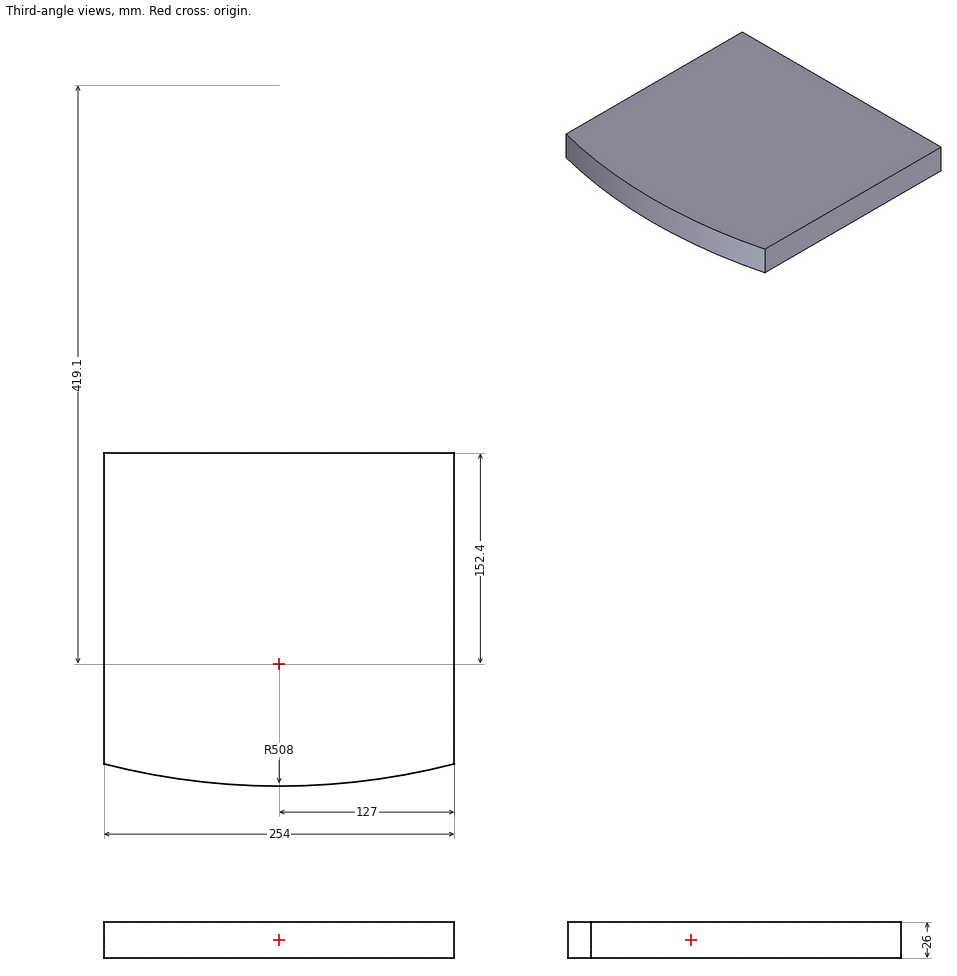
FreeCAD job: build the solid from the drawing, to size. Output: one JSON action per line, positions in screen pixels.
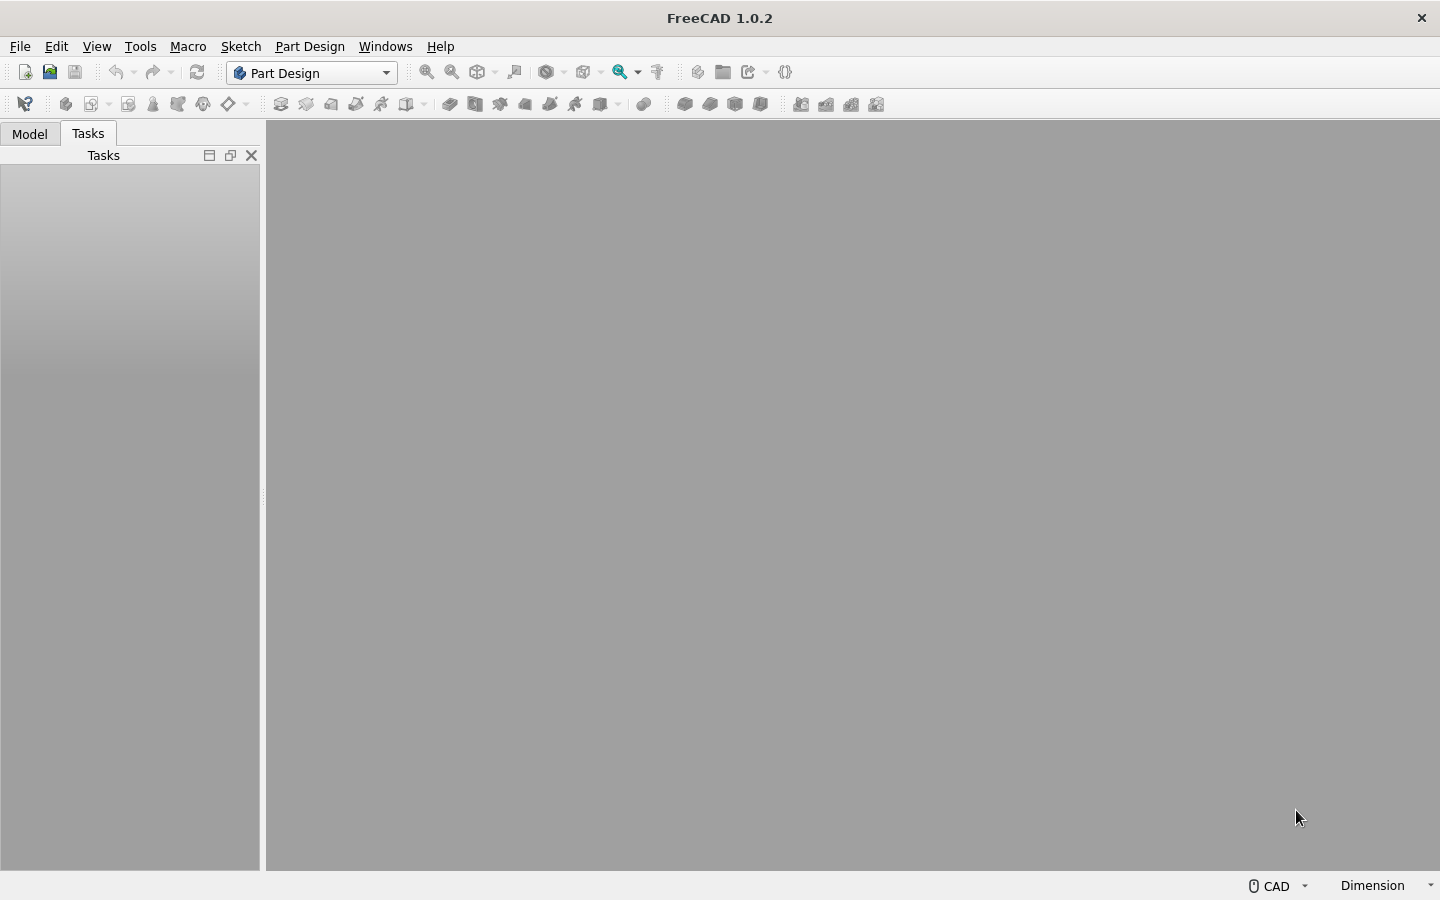
{"action": "left_click", "coordinate": [25, 72]}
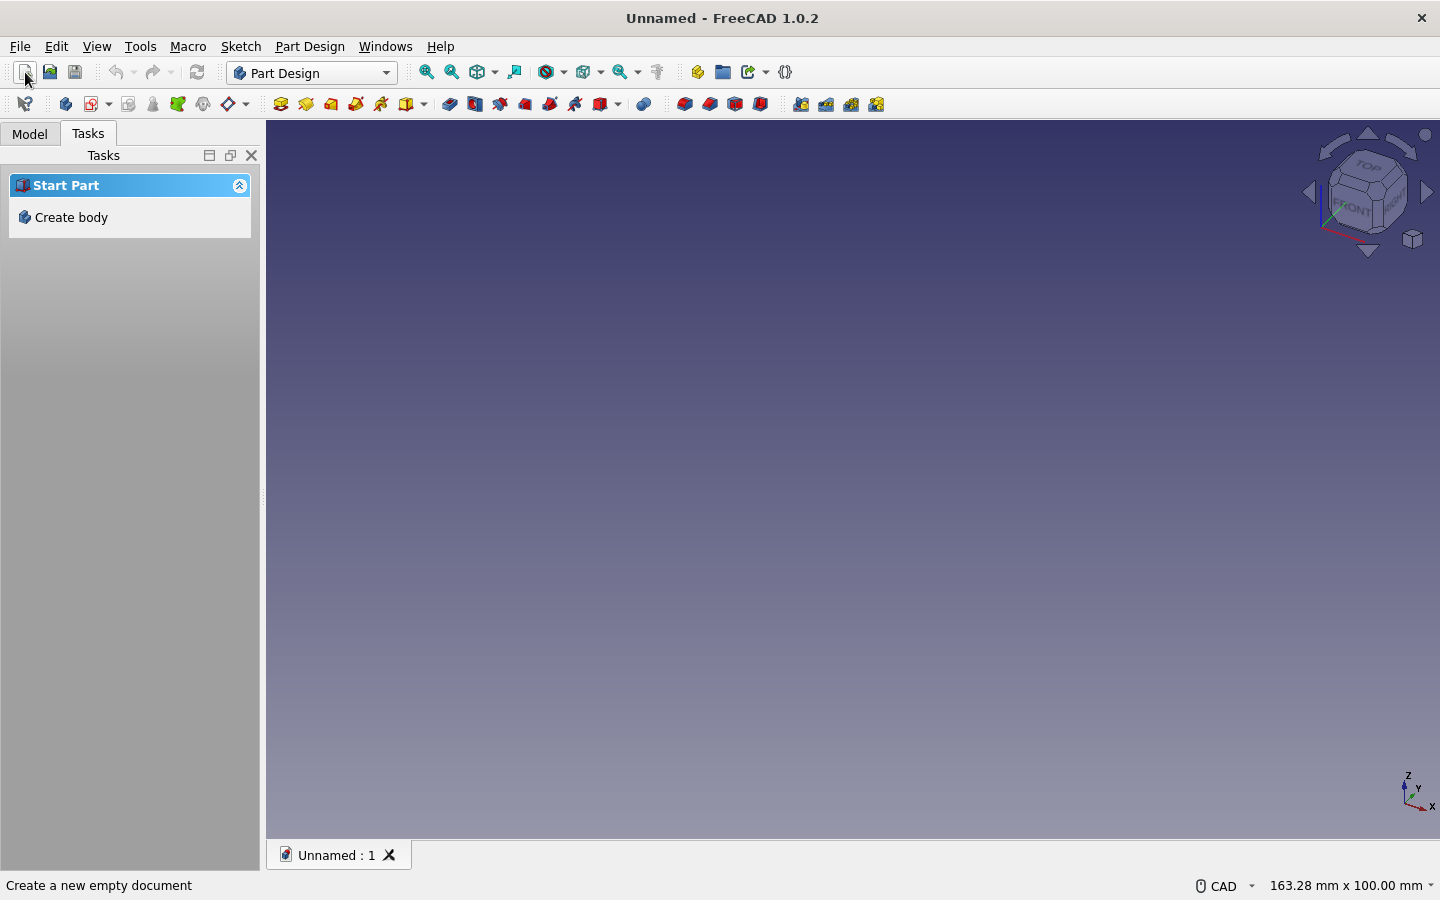
{"action": "left_click", "coordinate": [90, 104]}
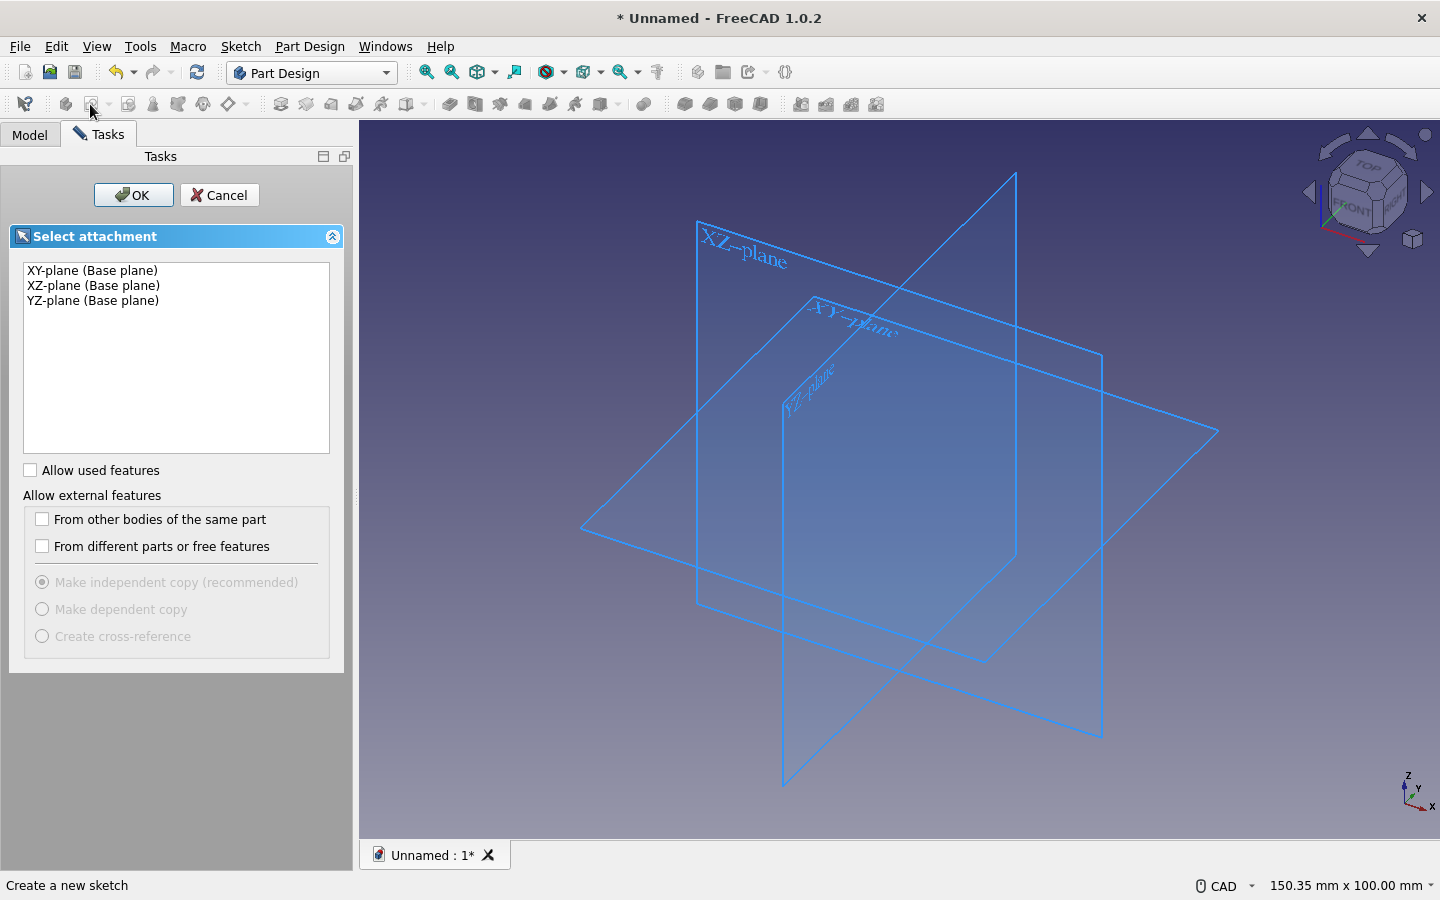
{"action": "left_click", "coordinate": [84, 270]}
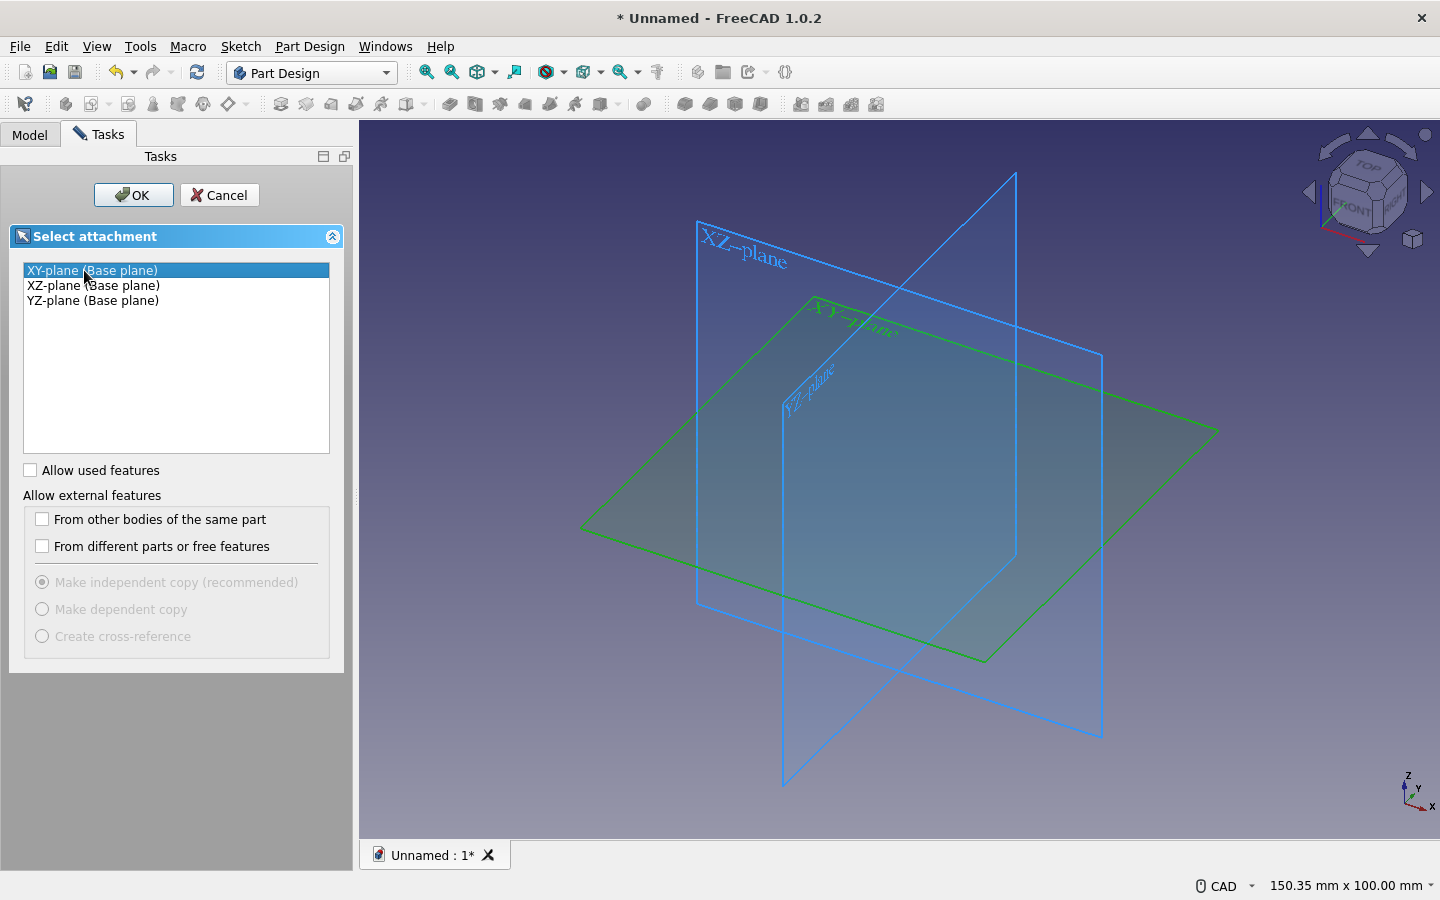
{"action": "left_click", "coordinate": [134, 195]}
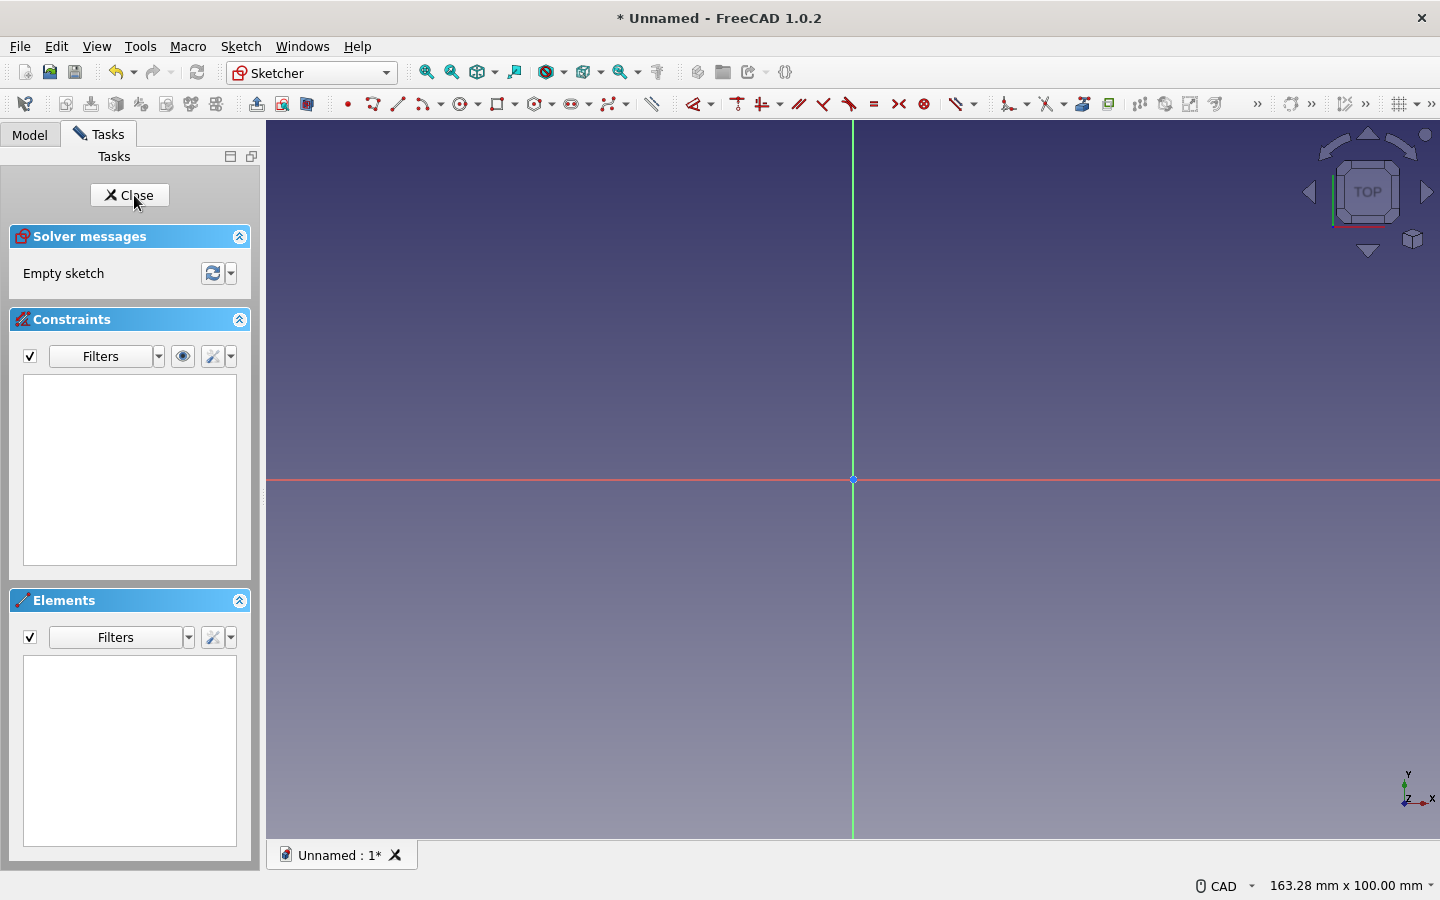
{"action": "scroll", "coordinate": [762, 554], "scroll_direction": "down", "scroll_amount": 7}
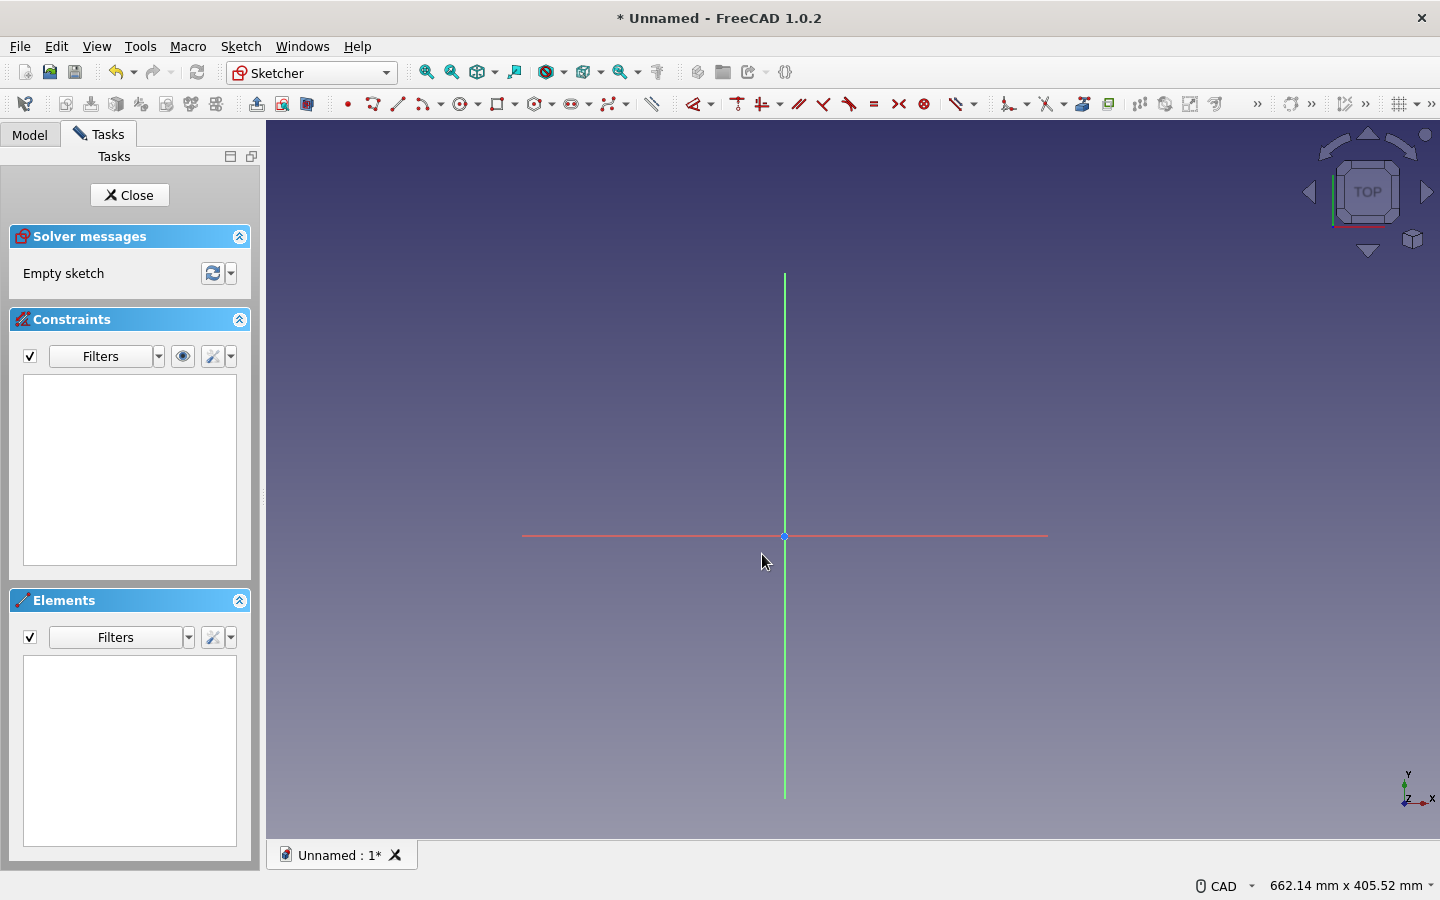
{"action": "left_click", "coordinate": [373, 104]}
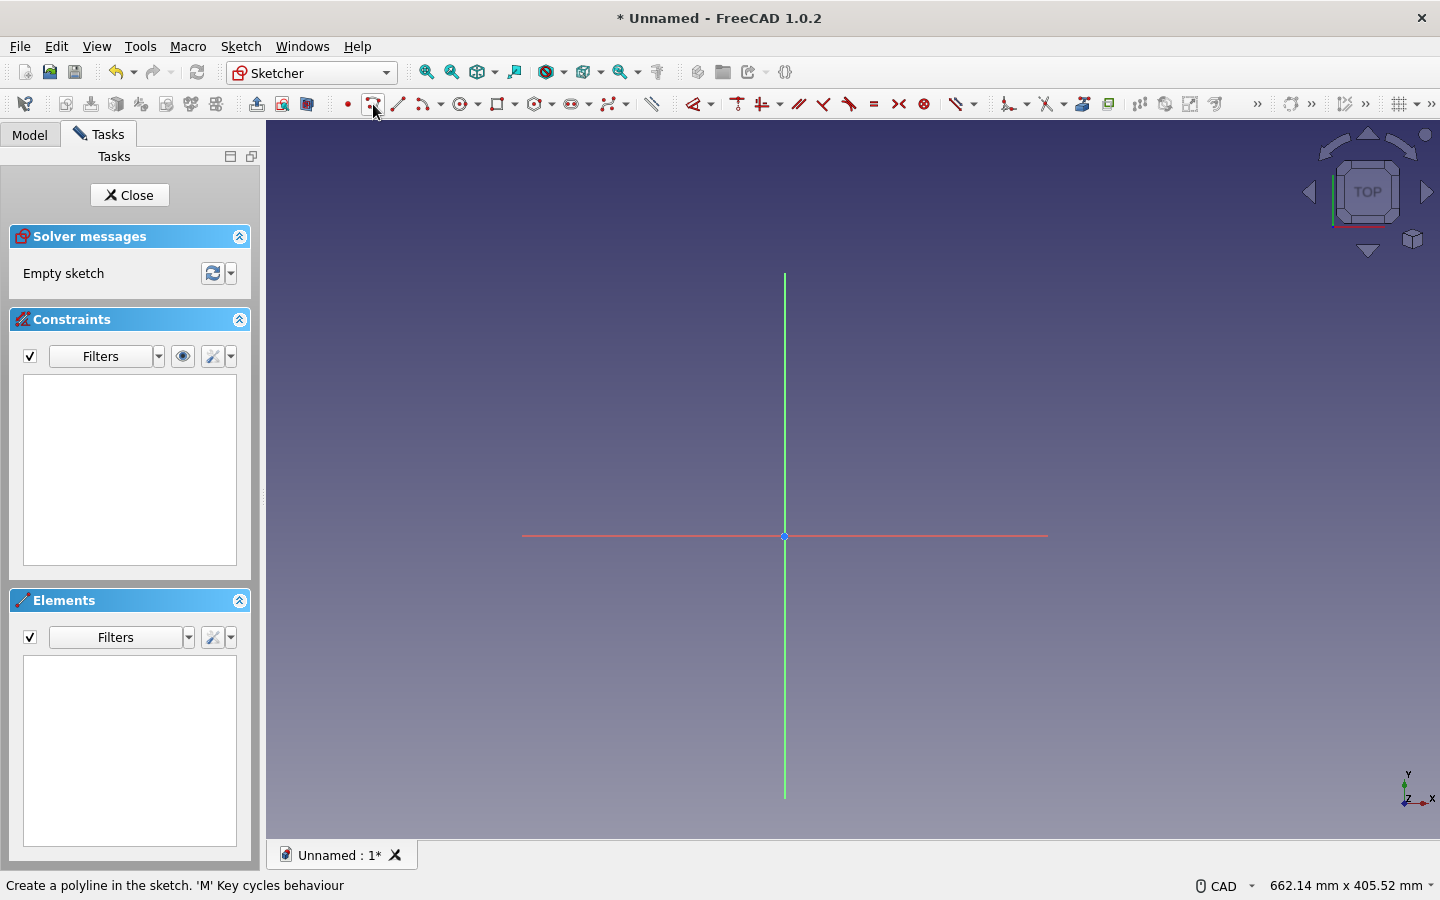
{"action": "left_click", "coordinate": [1010, 665]}
{"action": "left_click", "coordinate": [1010, 266]}
{"action": "left_click", "coordinate": [560, 266]}
{"action": "left_click", "coordinate": [560, 665]}
{"action": "right_click", "coordinate": [560, 665]}